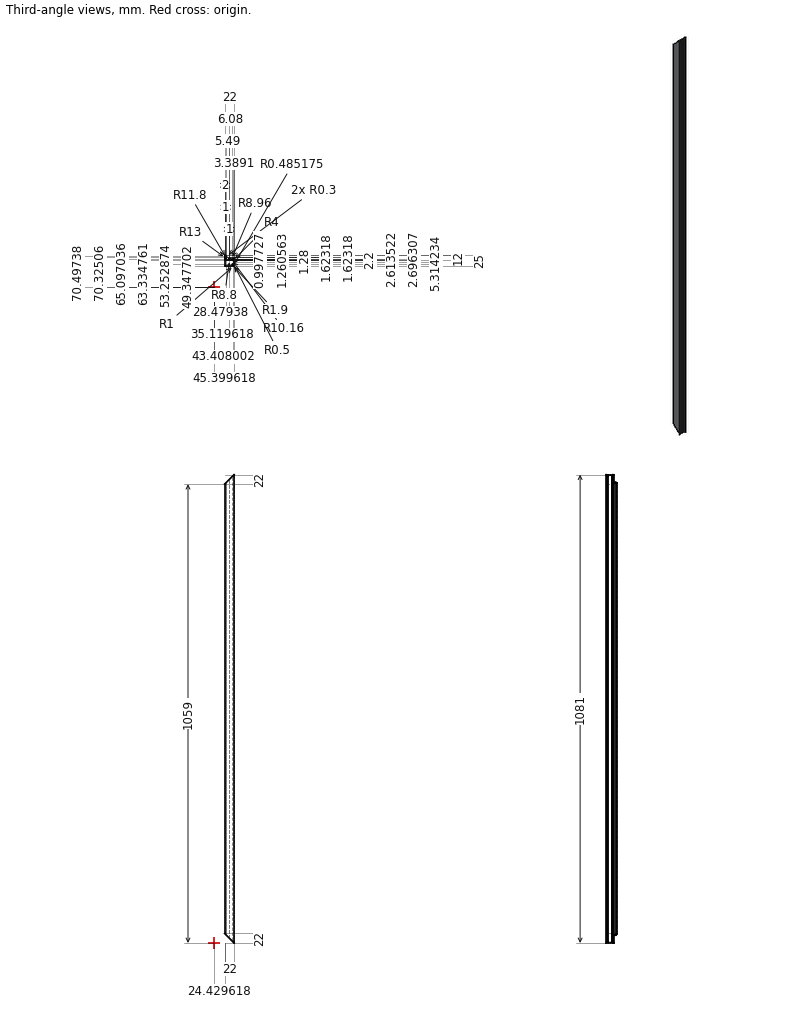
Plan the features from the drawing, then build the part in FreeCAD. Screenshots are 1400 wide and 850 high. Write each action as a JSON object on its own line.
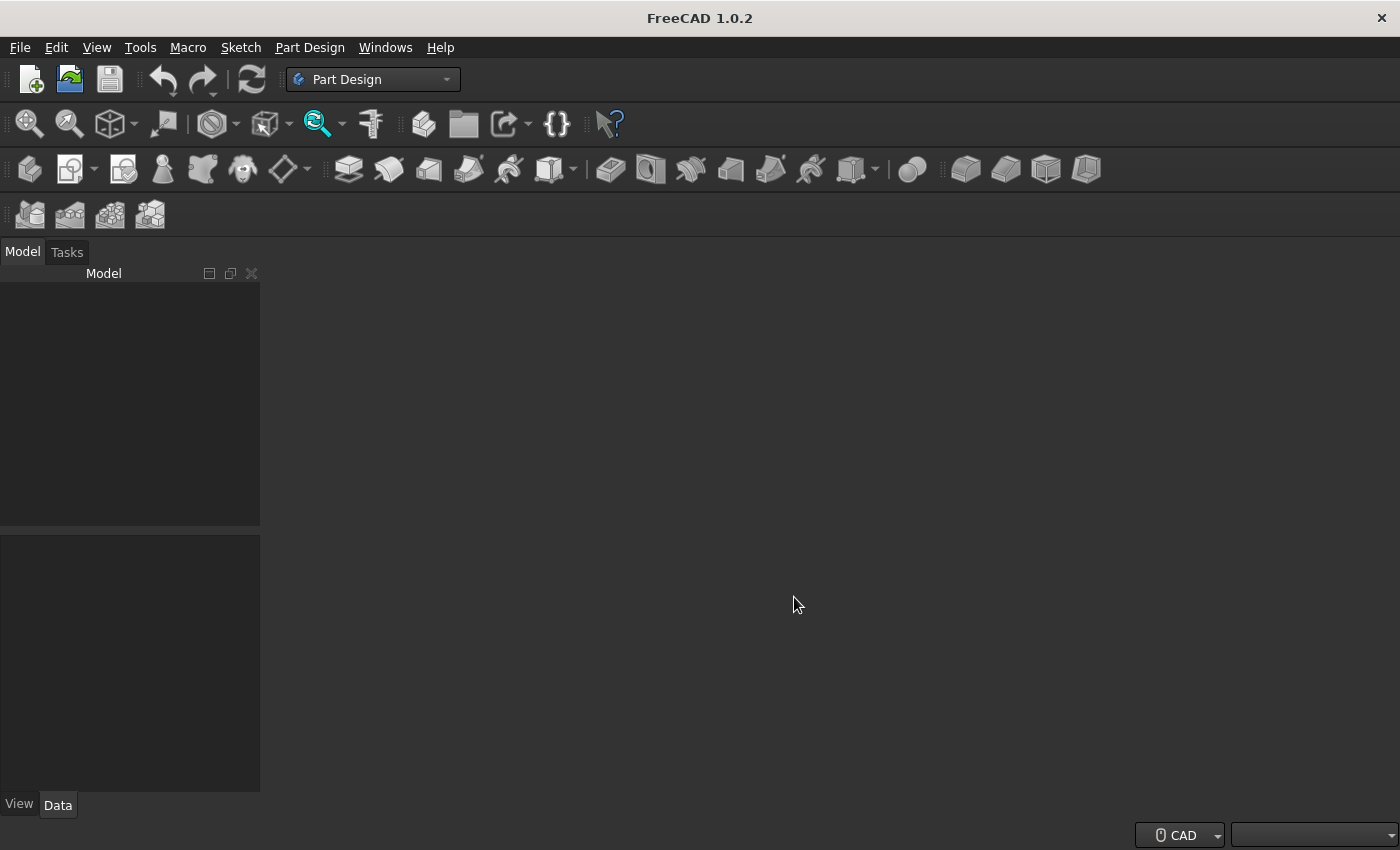
{"action": "left_click", "coordinate": [30, 80]}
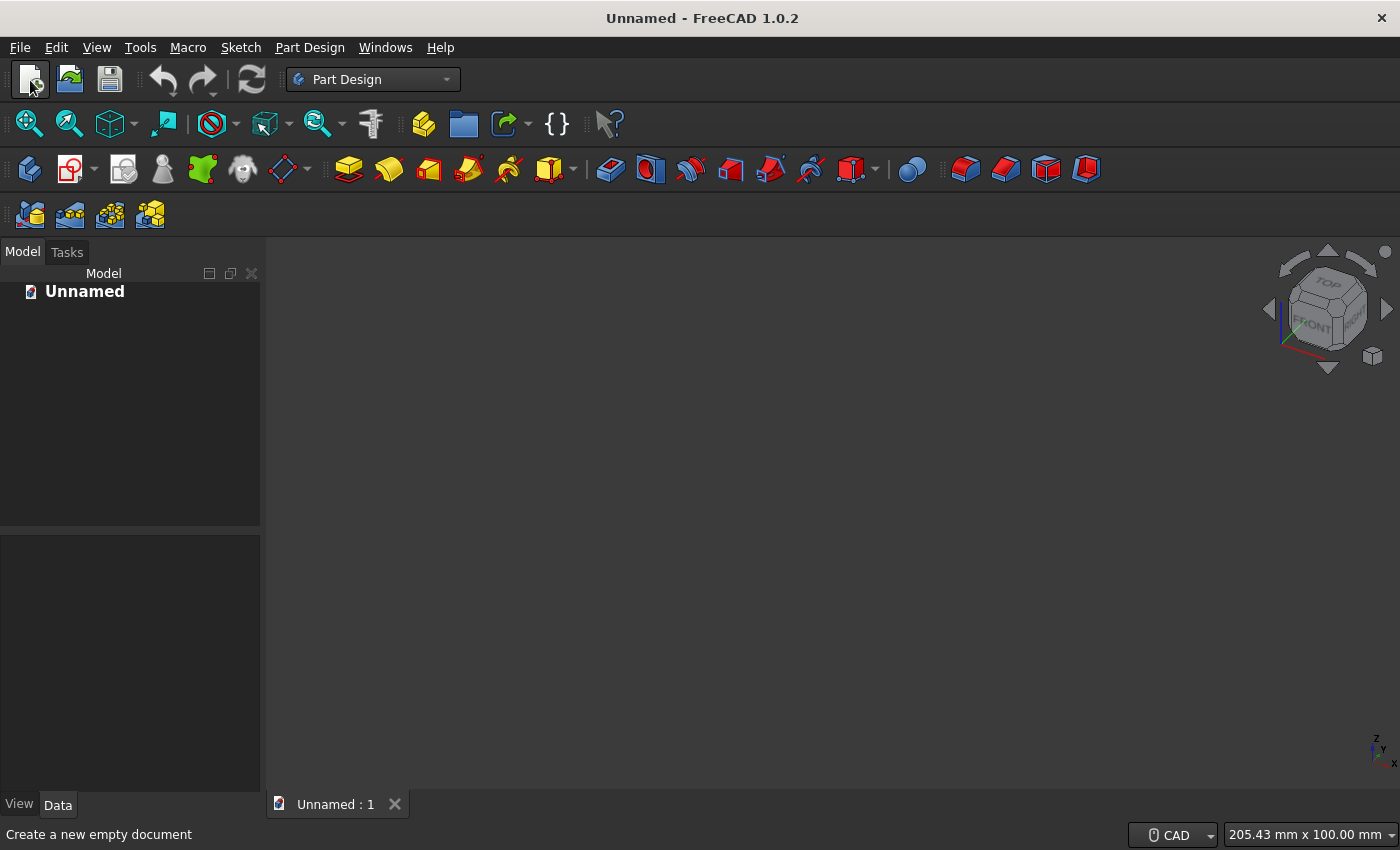
{"action": "left_click", "coordinate": [70, 170]}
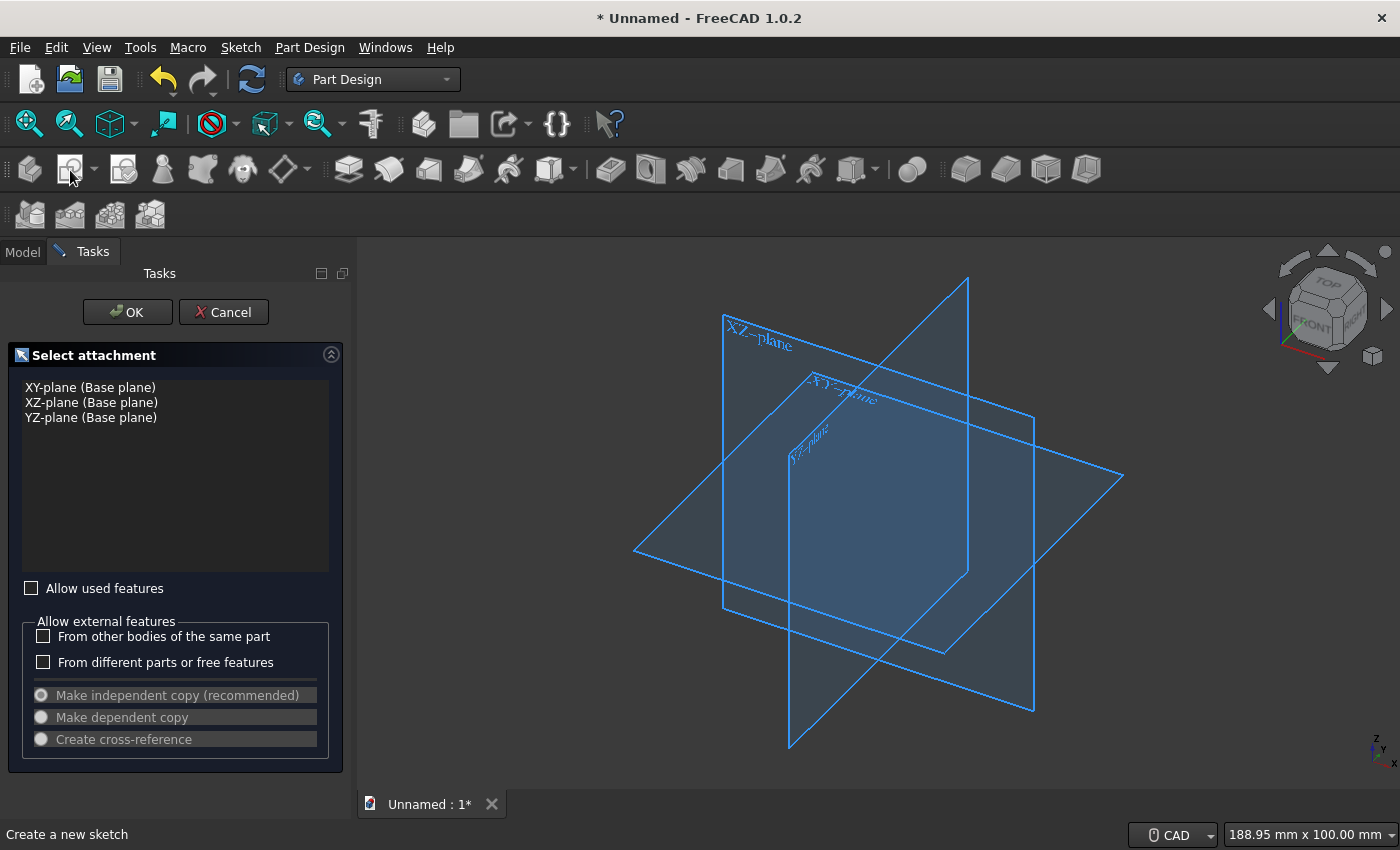
{"action": "left_click", "coordinate": [82, 388]}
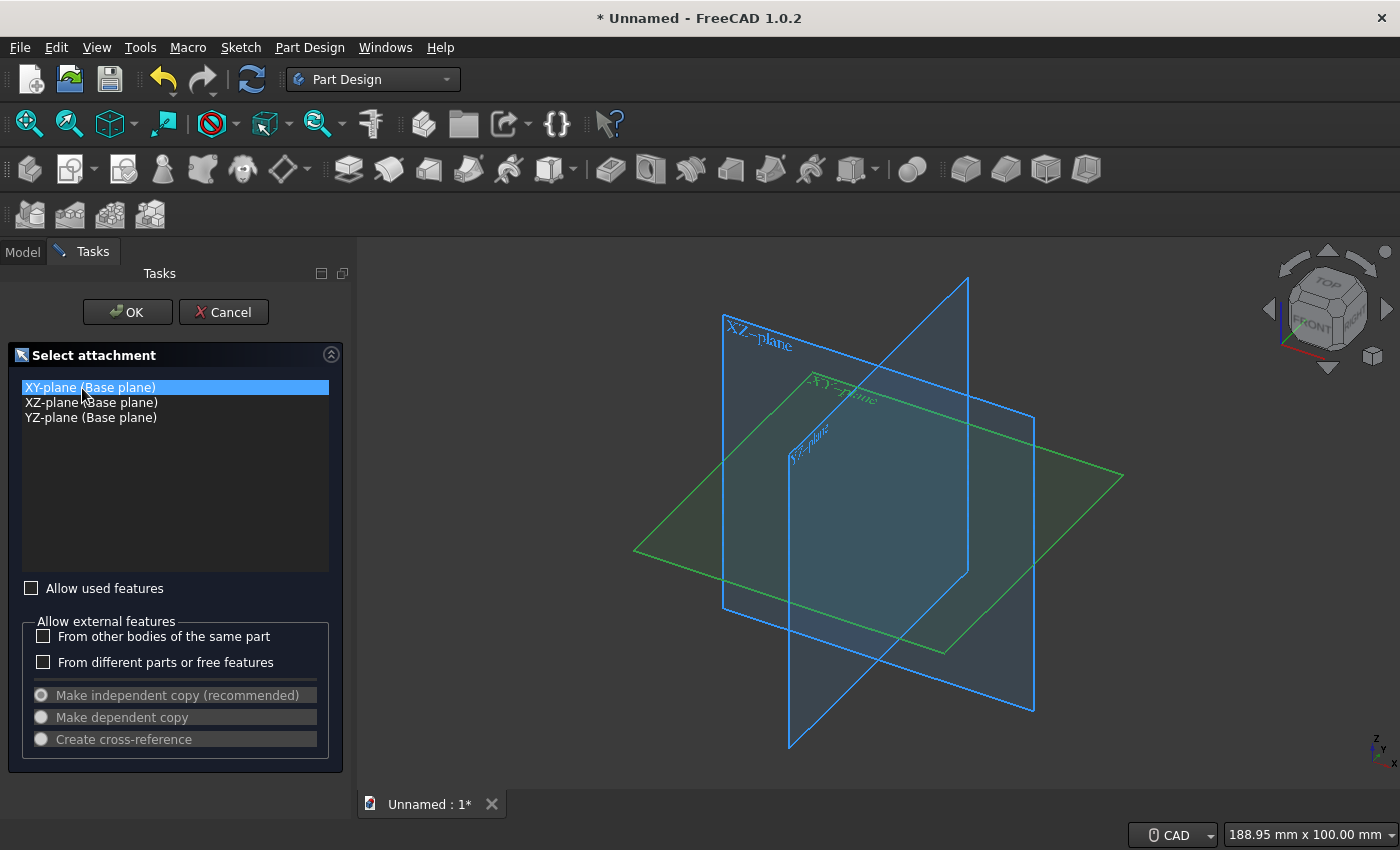
{"action": "left_click", "coordinate": [128, 312]}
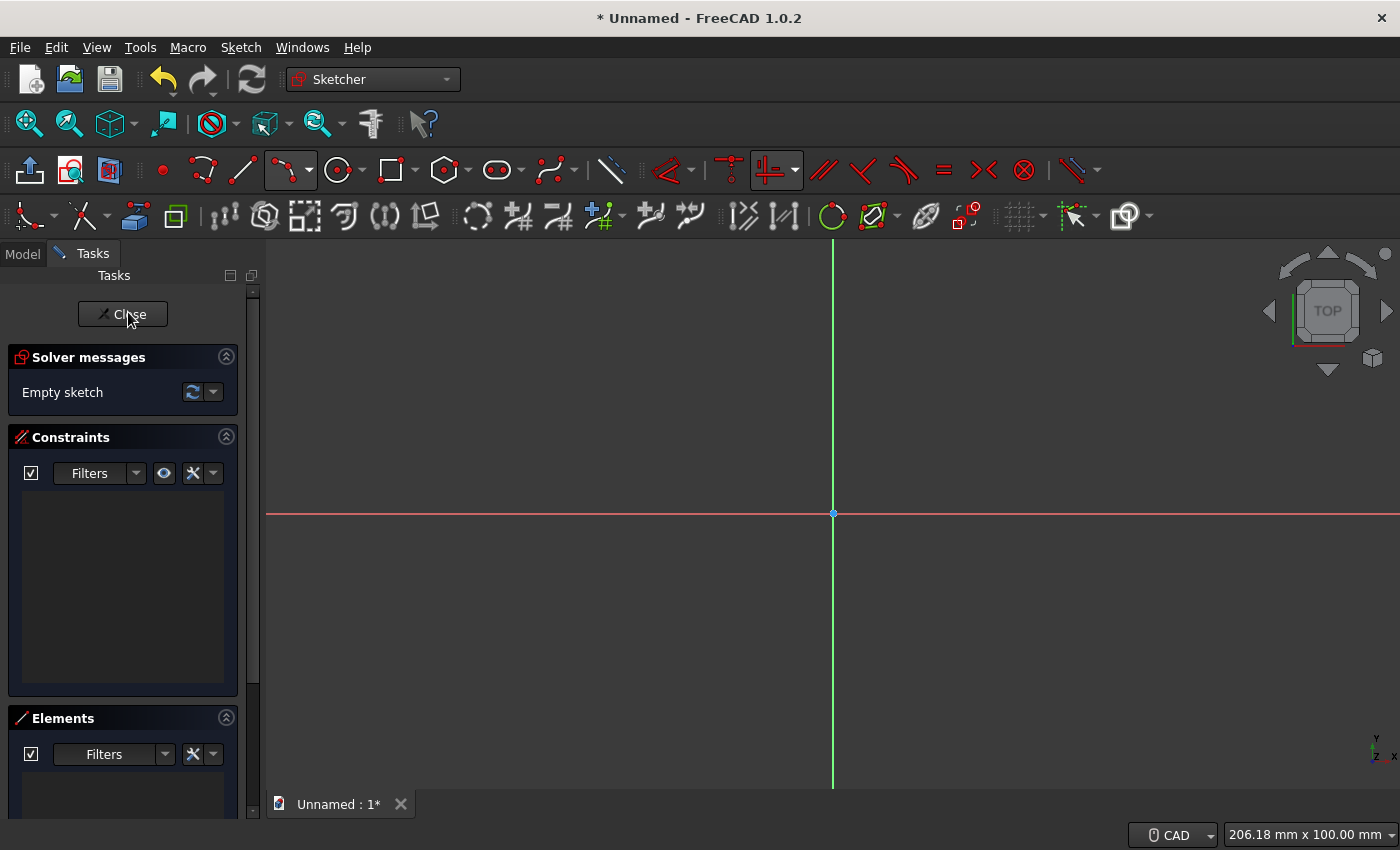
{"action": "scroll", "coordinate": [764, 514], "scroll_direction": "down", "scroll_amount": 5}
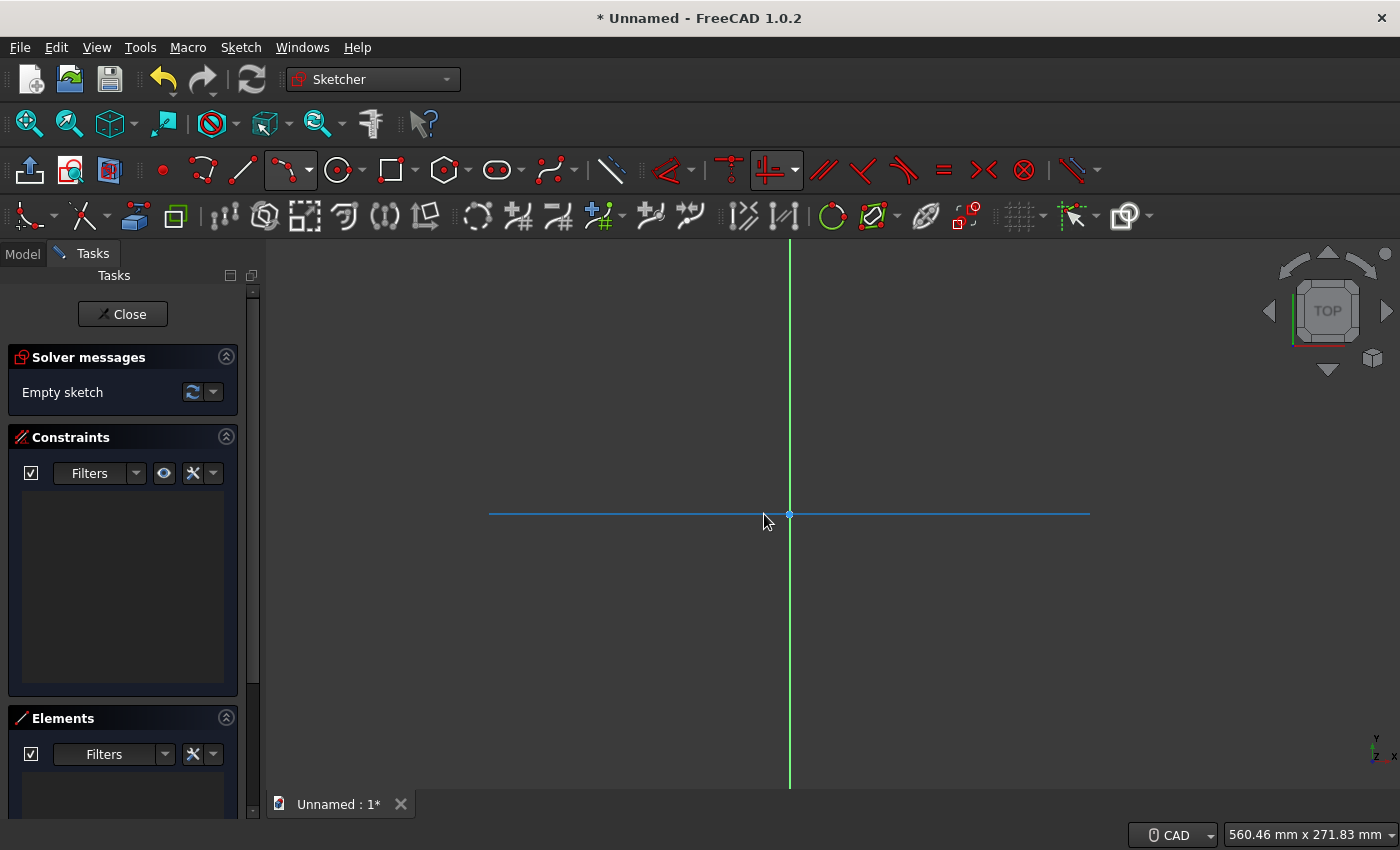
{"action": "scroll", "coordinate": [877, 372], "scroll_direction": "up", "scroll_amount": 10}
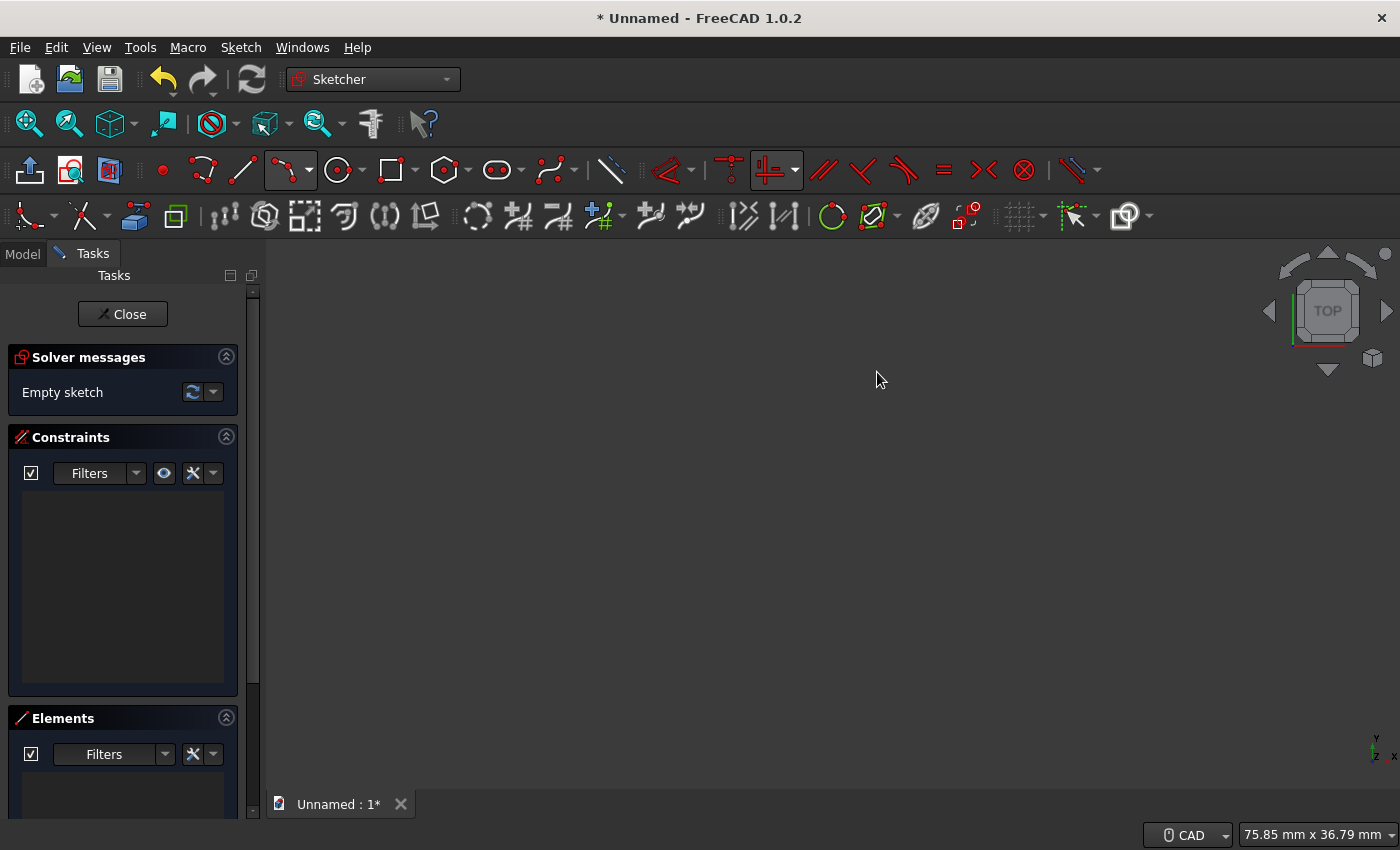
{"action": "left_click", "coordinate": [244, 170]}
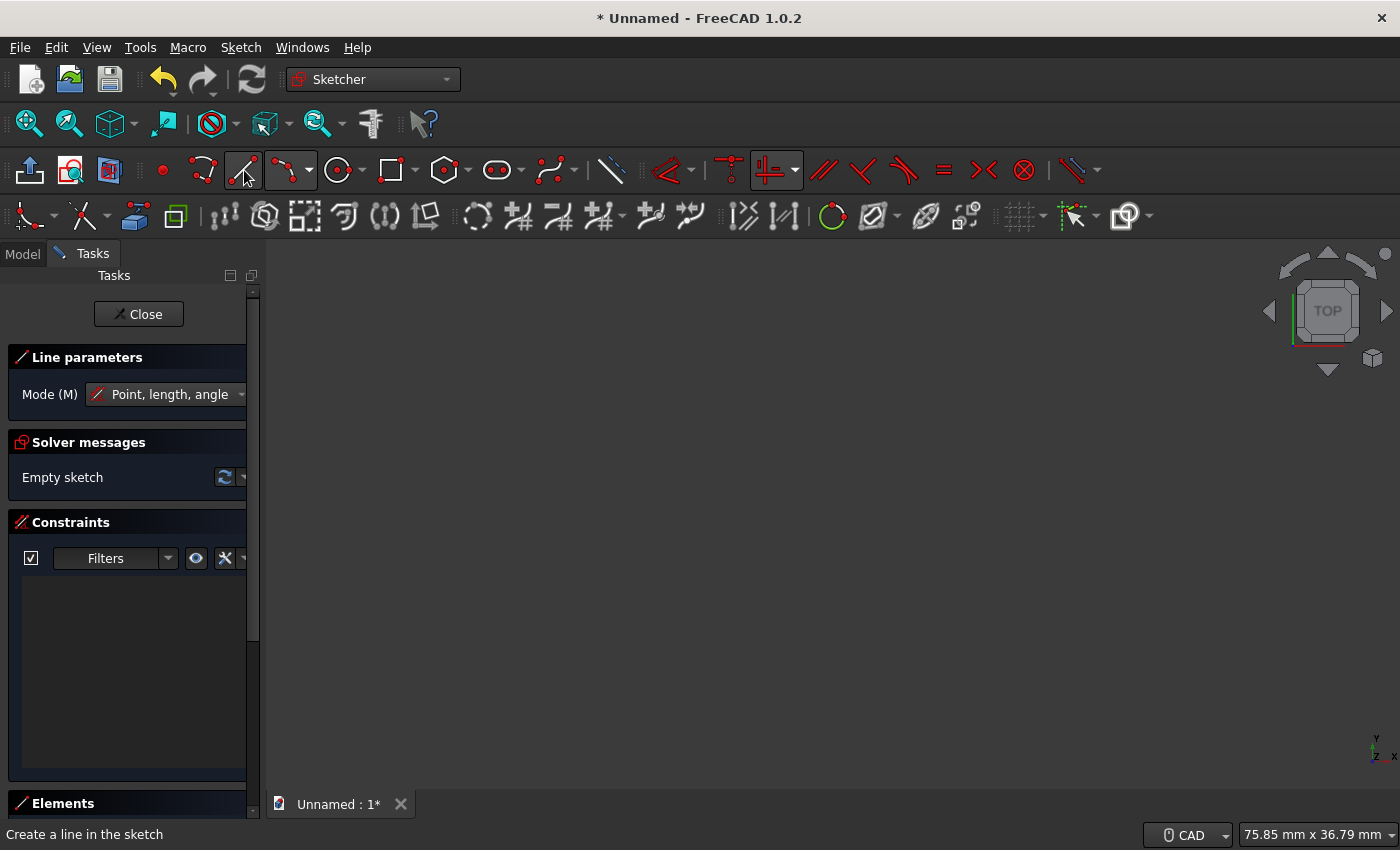
{"action": "left_click", "coordinate": [907, 626]}
{"action": "left_click", "coordinate": [907, 546]}